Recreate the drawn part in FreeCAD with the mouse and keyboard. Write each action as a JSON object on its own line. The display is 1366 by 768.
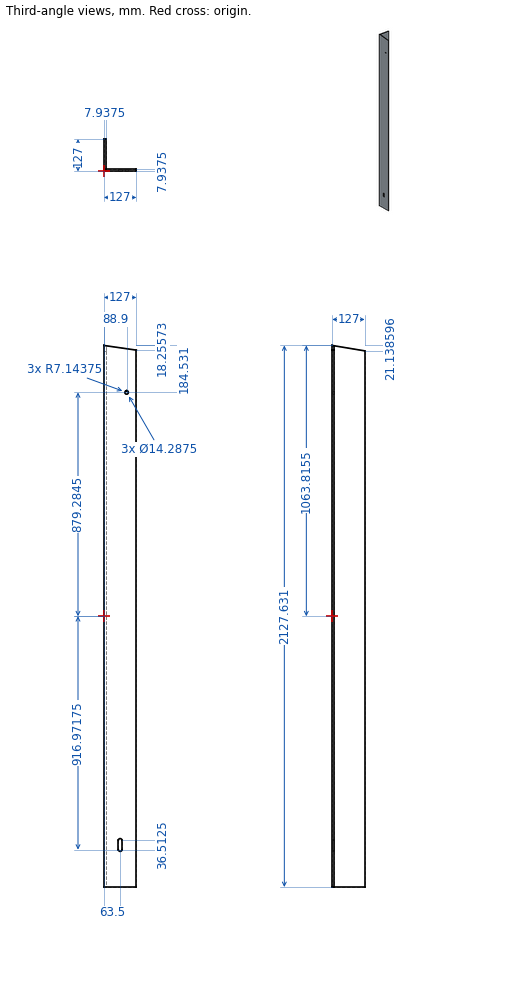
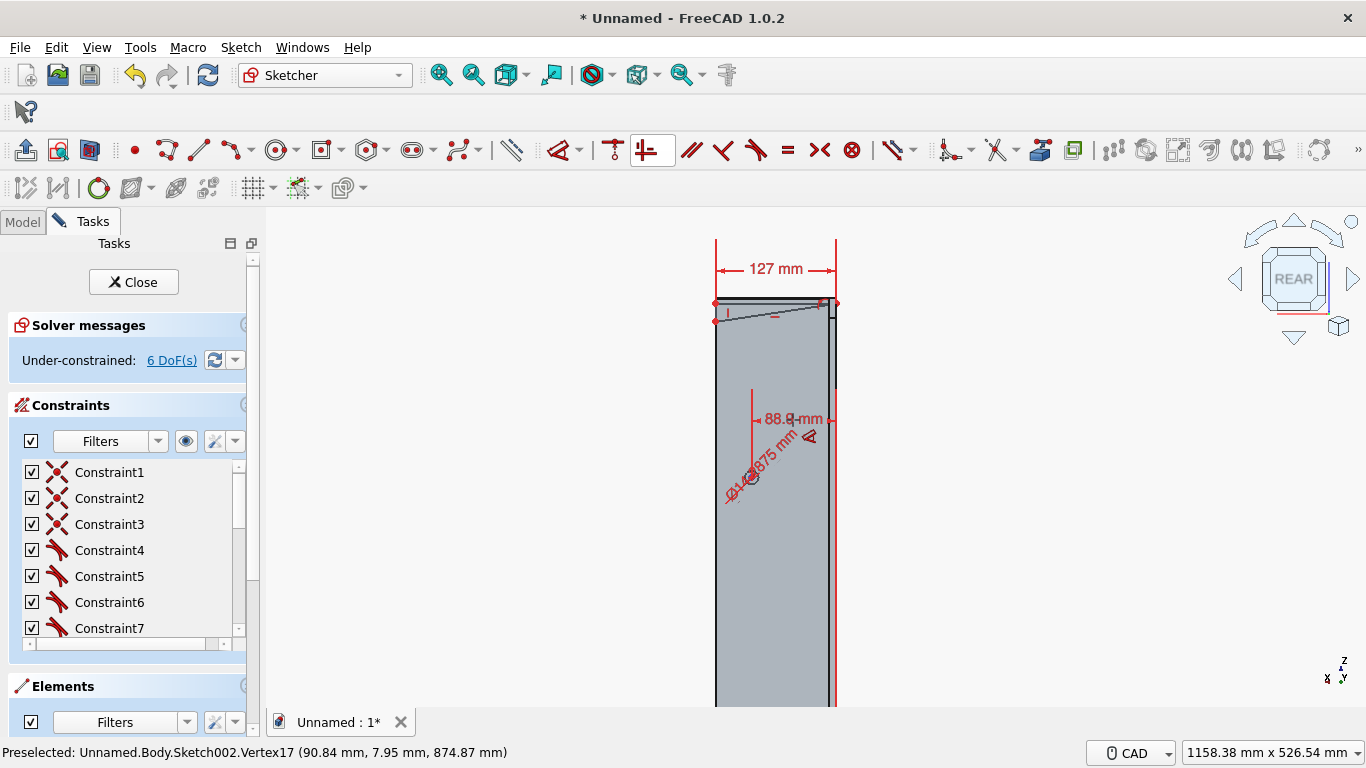
{"action": "scroll", "coordinate": [742, 302], "scroll_direction": "down", "scroll_amount": 9}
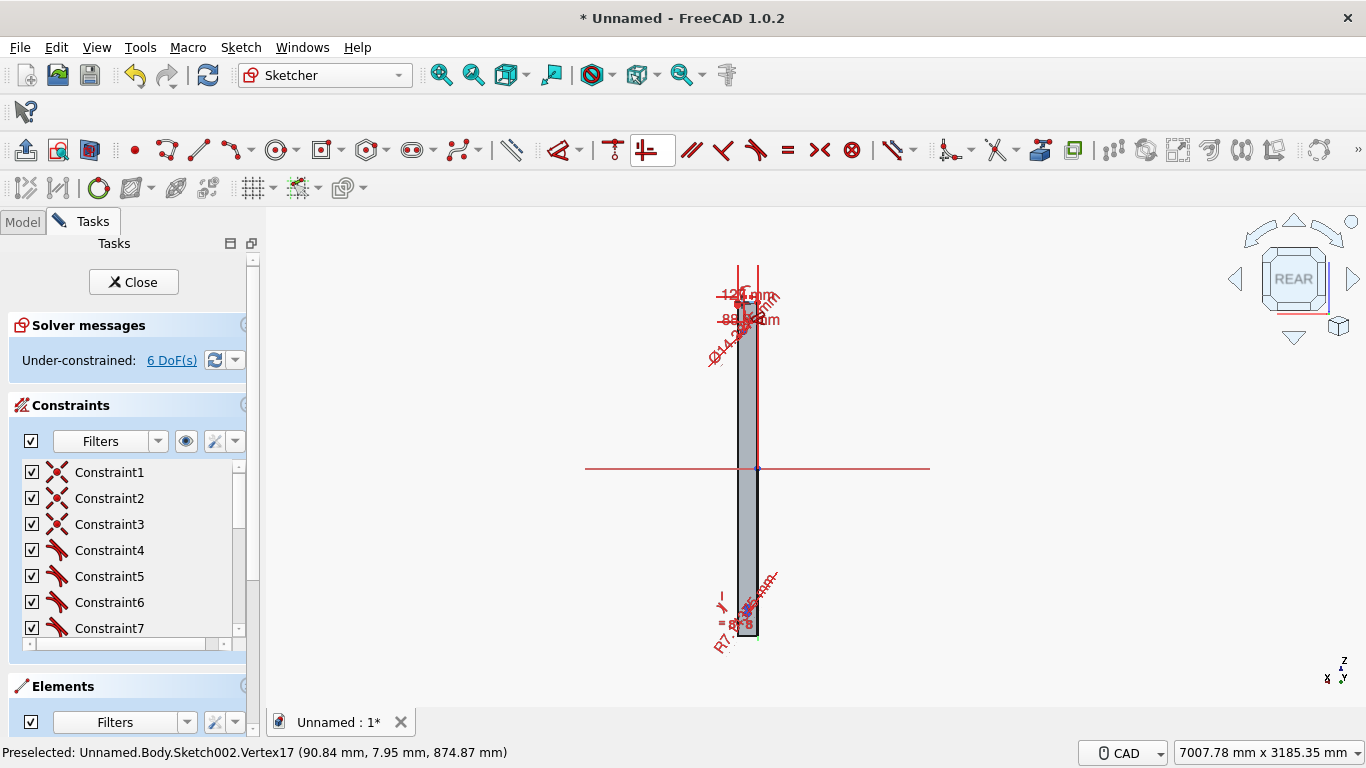
{"action": "scroll", "coordinate": [748, 613], "scroll_direction": "up", "scroll_amount": 12}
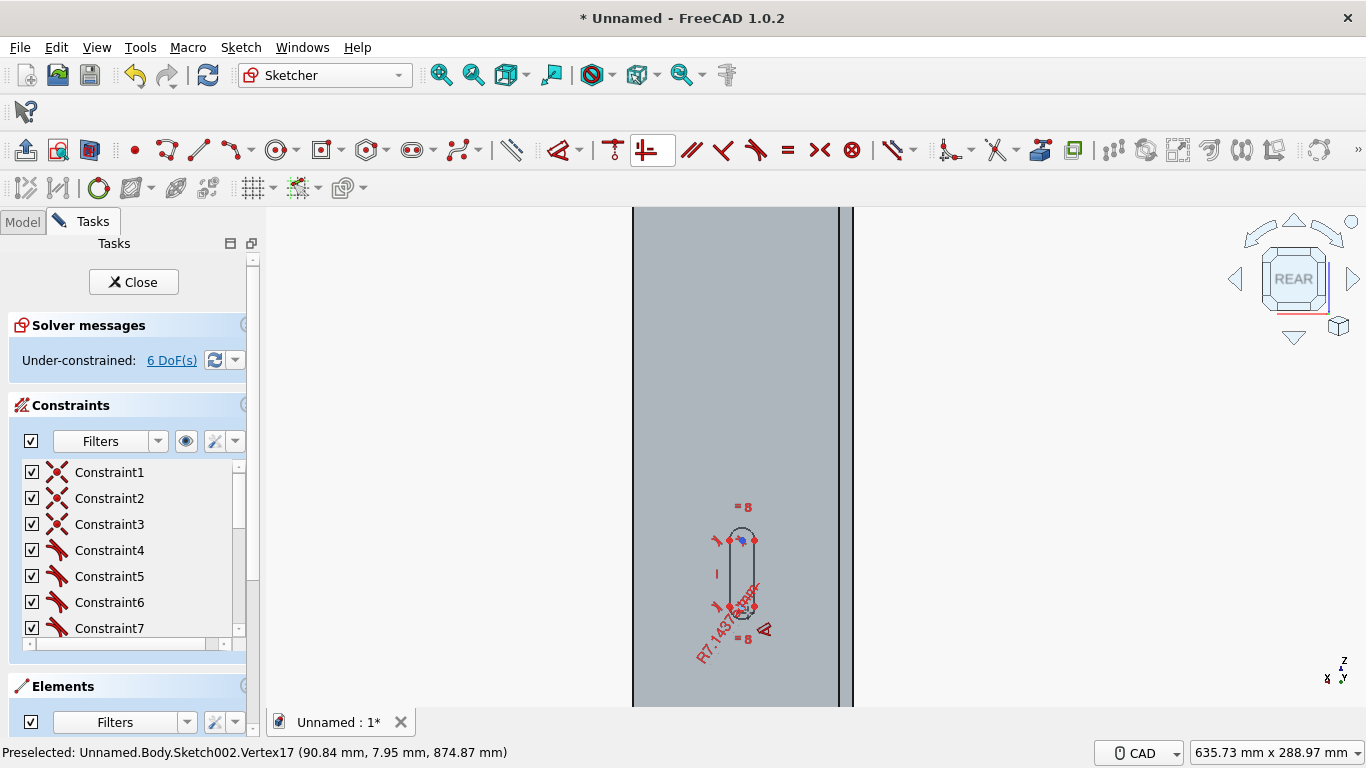
{"action": "left_click", "coordinate": [742, 607]}
{"action": "left_click", "coordinate": [823, 641]}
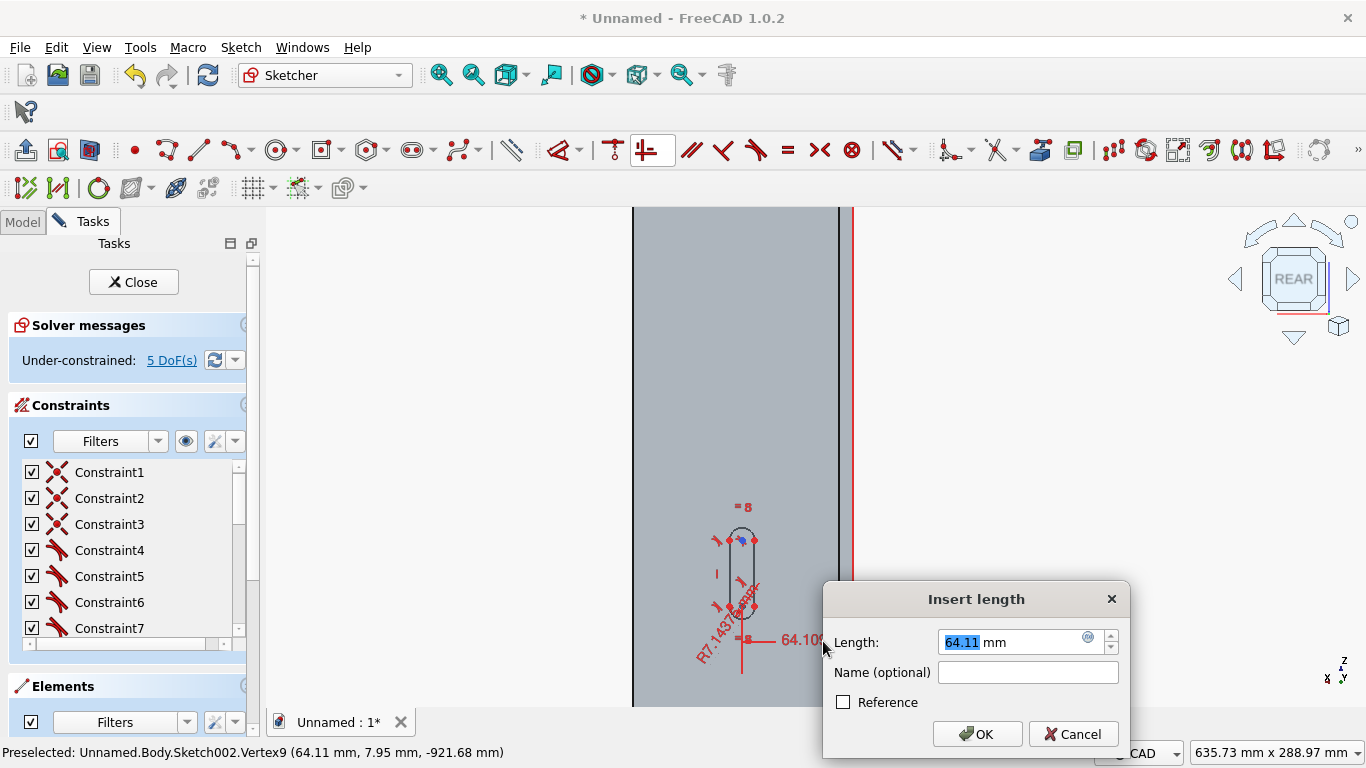
{"action": "type", "text": "63.5"}
{"action": "key", "text": "Return"}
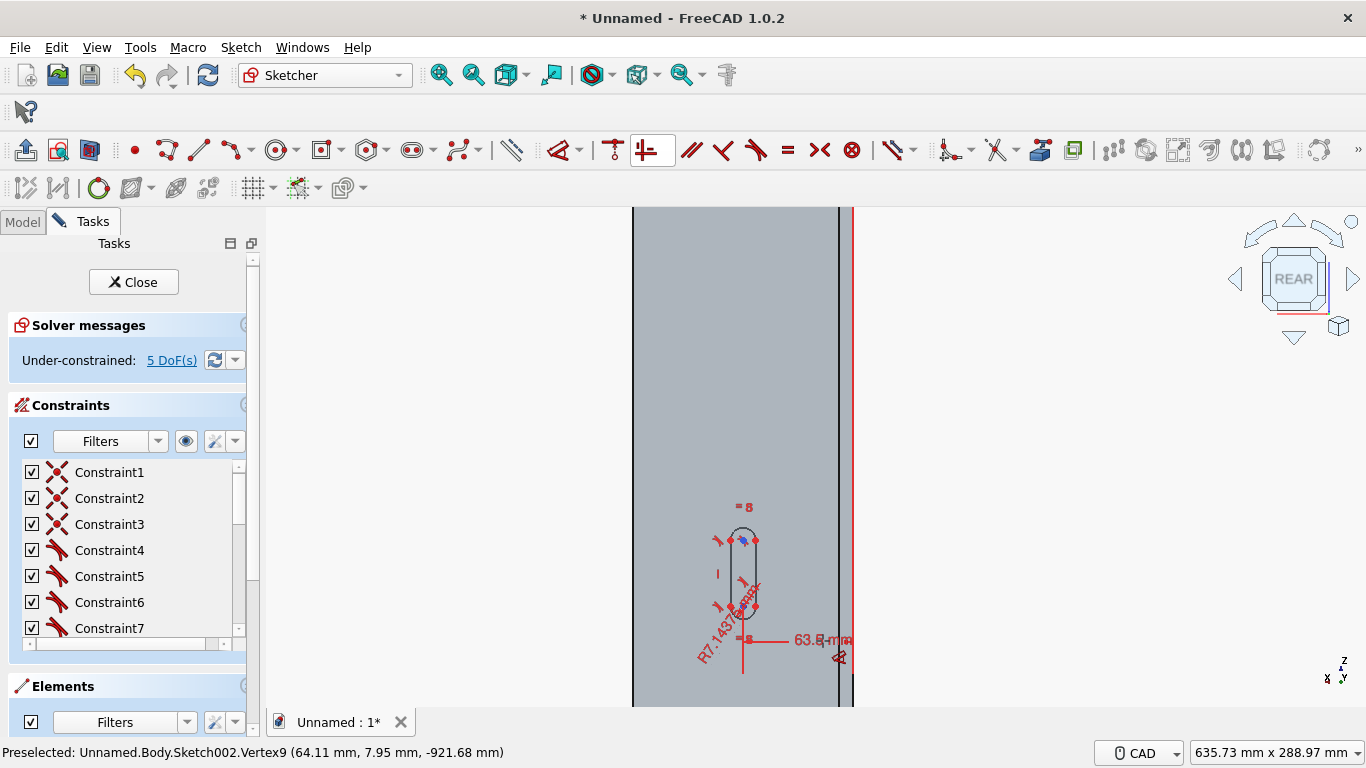
{"action": "left_click", "coordinate": [731, 587]}
{"action": "left_click", "coordinate": [697, 574]}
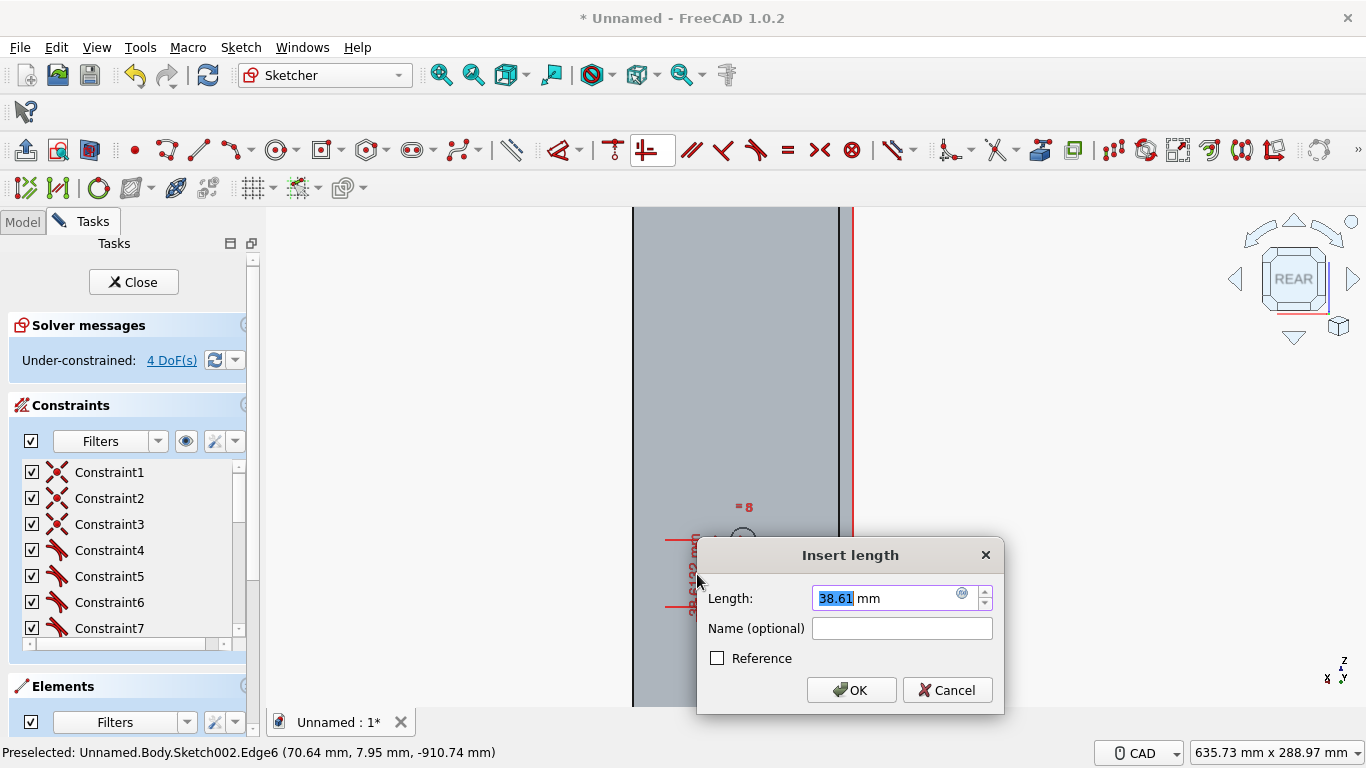
{"action": "type", "text": "36.5125"}
{"action": "key", "text": "Return"}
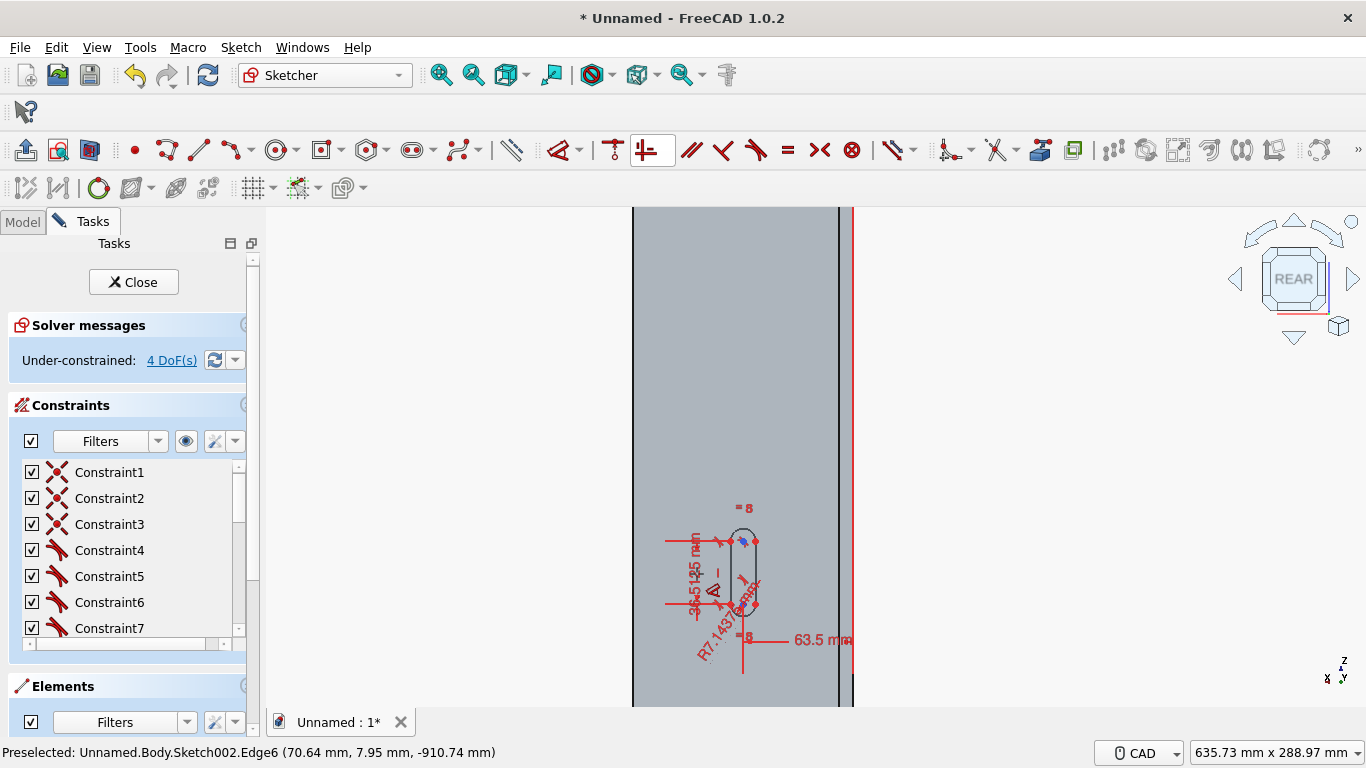
{"action": "scroll", "coordinate": [748, 613], "scroll_direction": "down", "scroll_amount": 12}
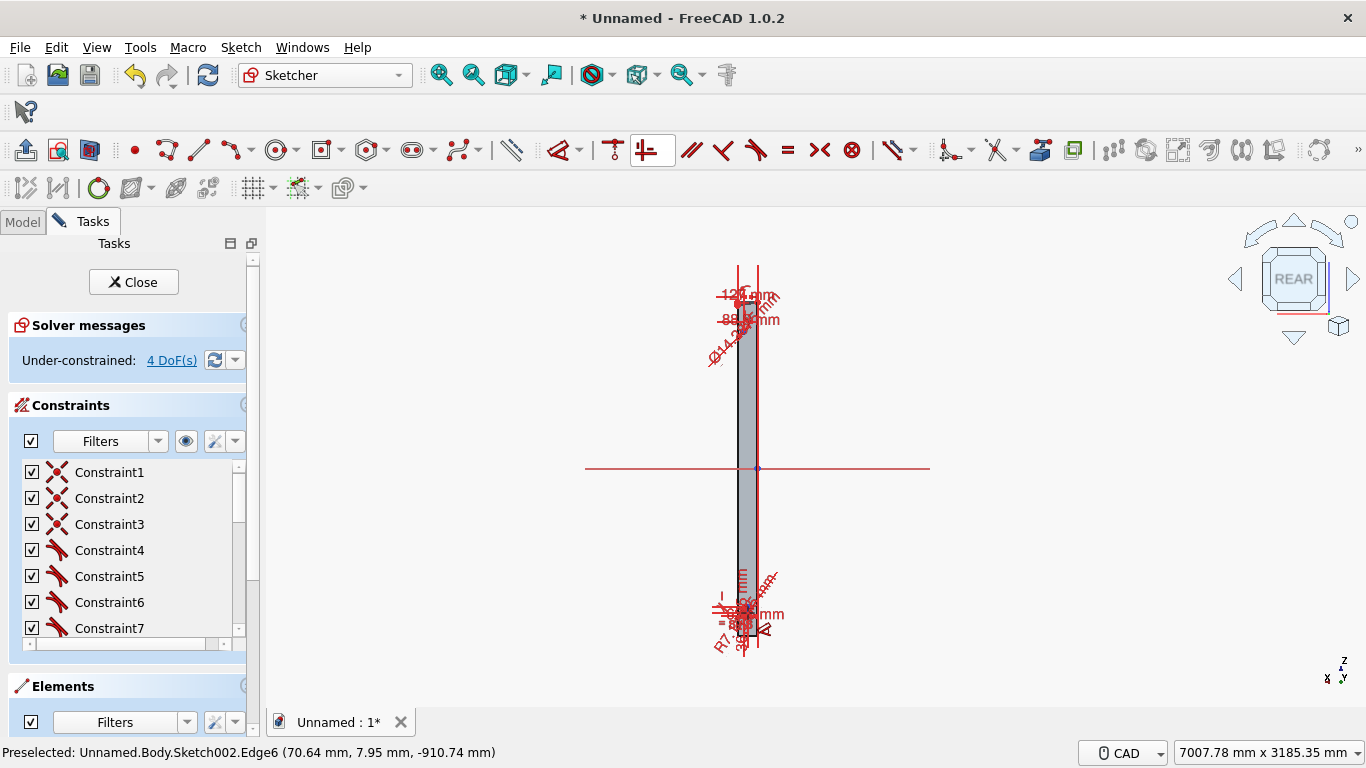
{"action": "scroll", "coordinate": [738, 303], "scroll_direction": "up", "scroll_amount": 14}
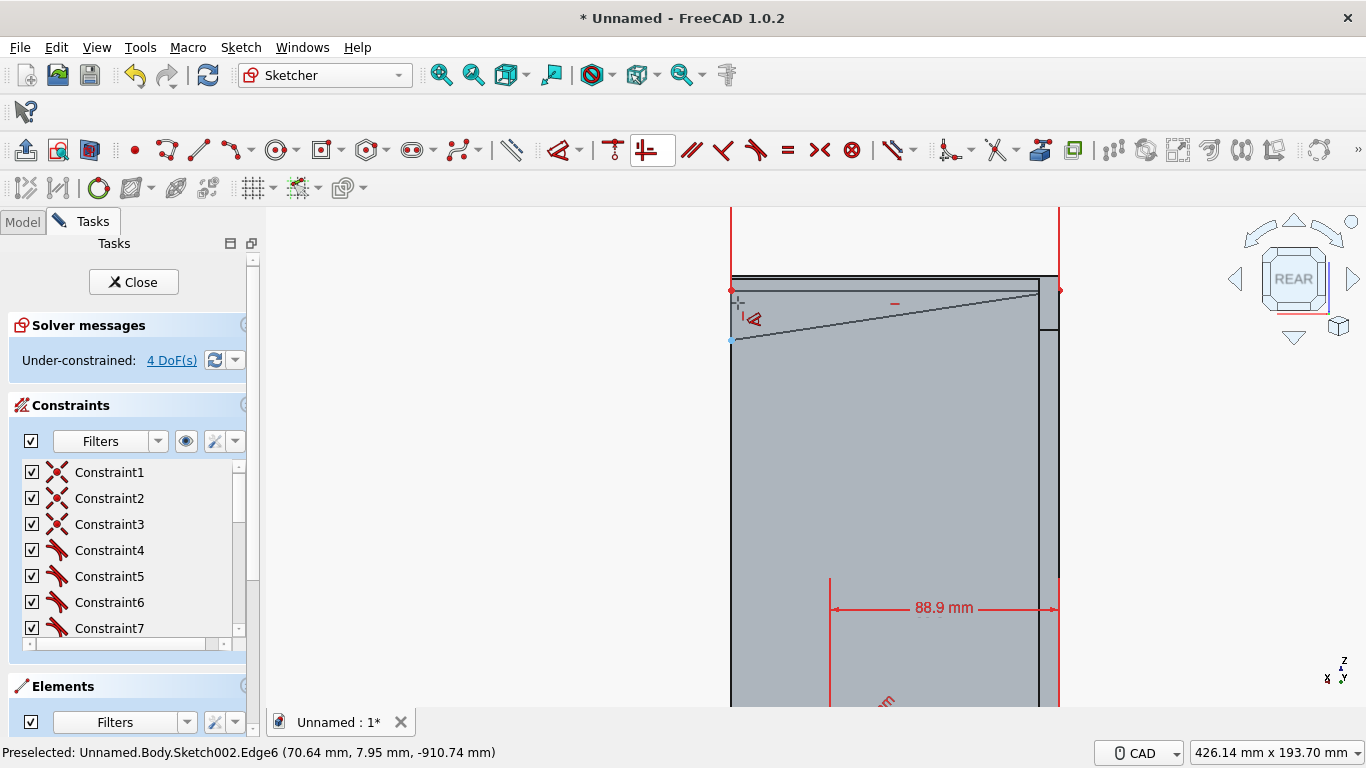
{"action": "left_click", "coordinate": [731, 306]}
{"action": "left_click", "coordinate": [697, 316]}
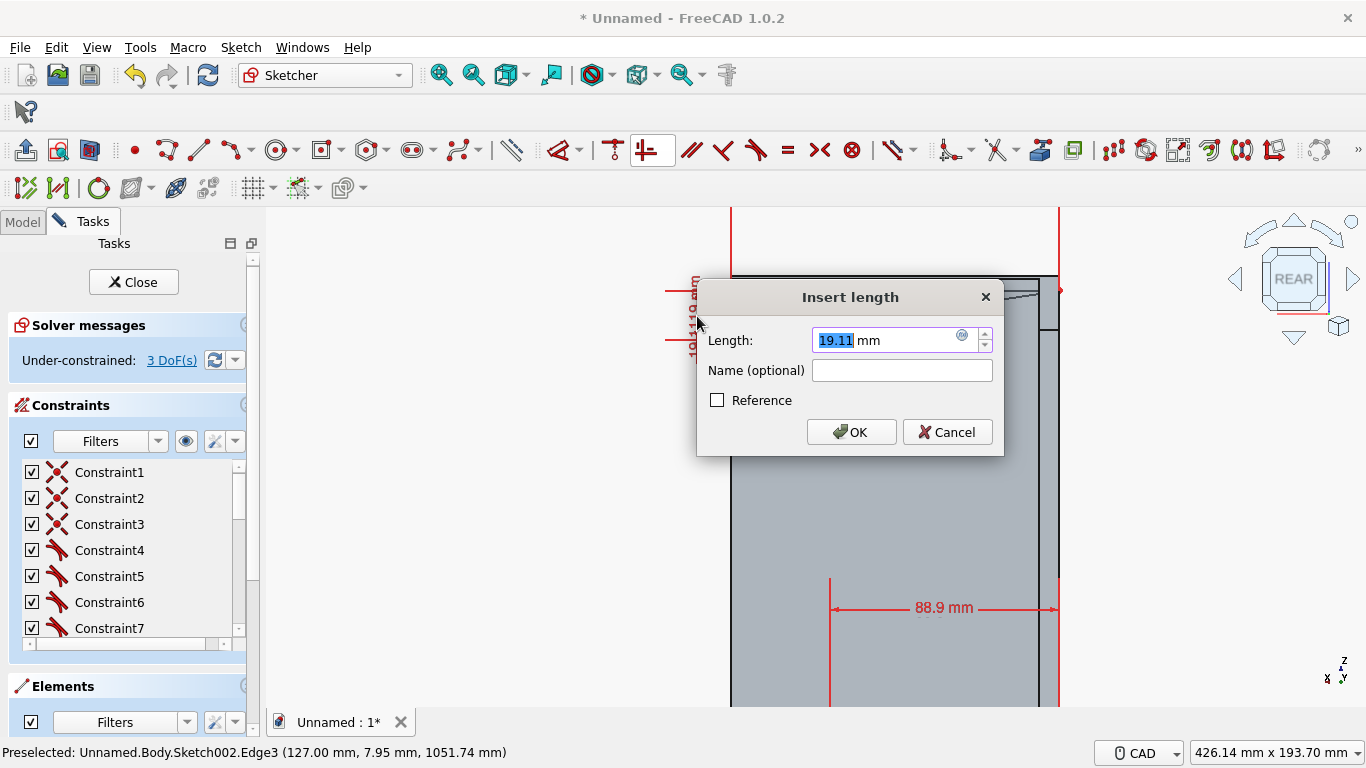
{"action": "type", "text": "18.25573"}
{"action": "key", "text": "Return"}